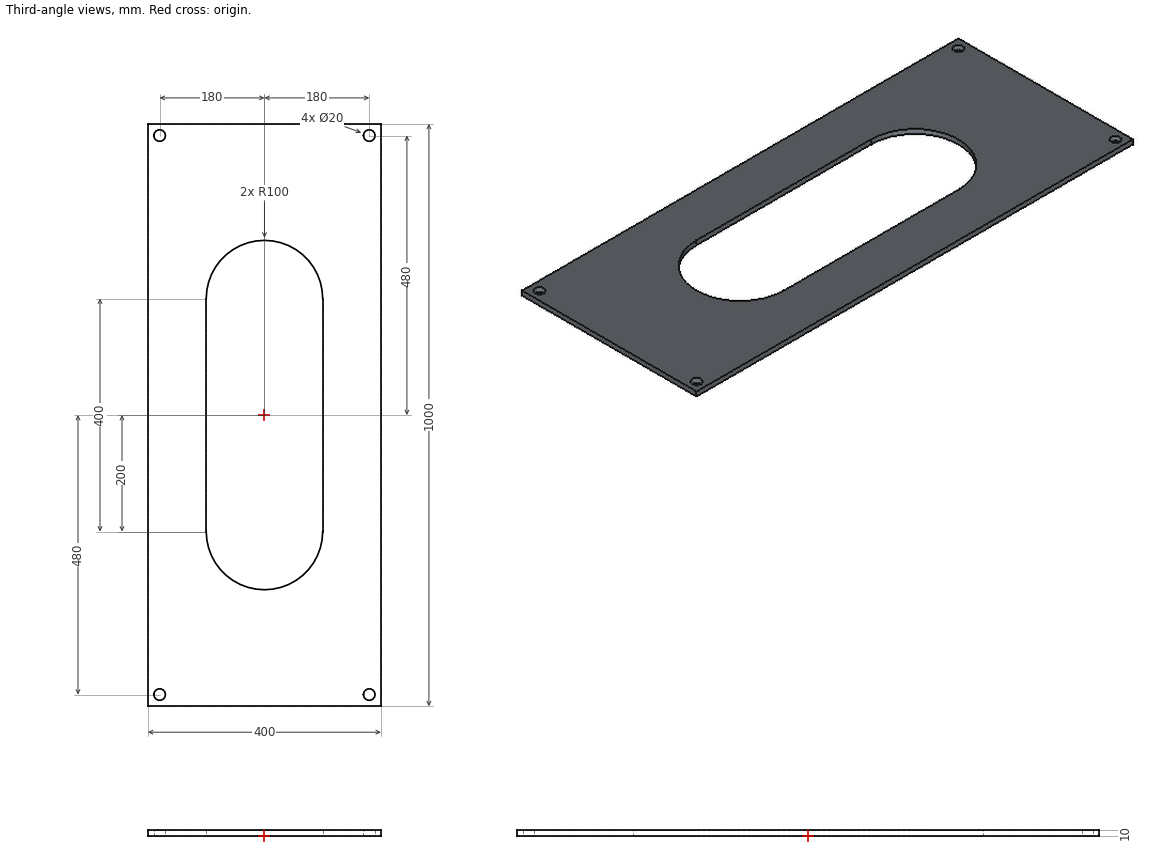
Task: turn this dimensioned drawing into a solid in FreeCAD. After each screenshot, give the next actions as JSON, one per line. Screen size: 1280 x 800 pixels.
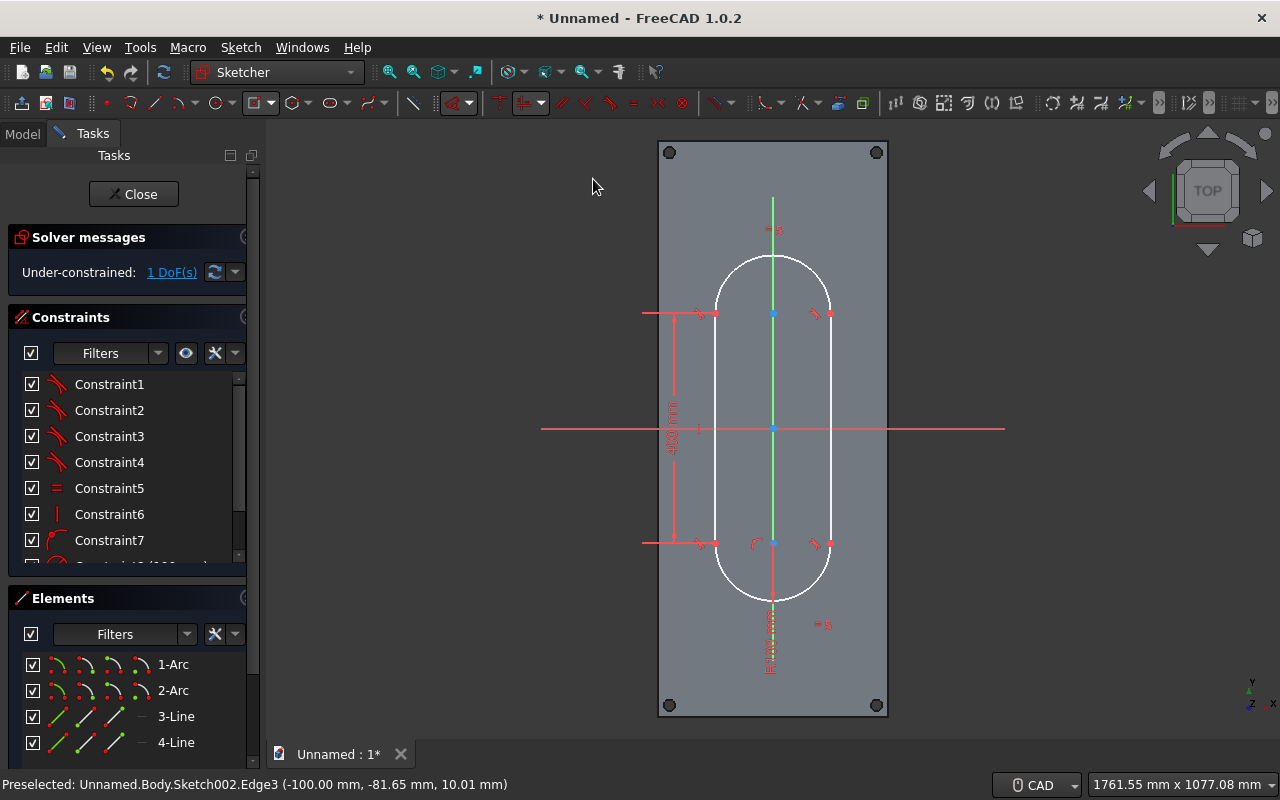
{"action": "left_click", "coordinate": [715, 543]}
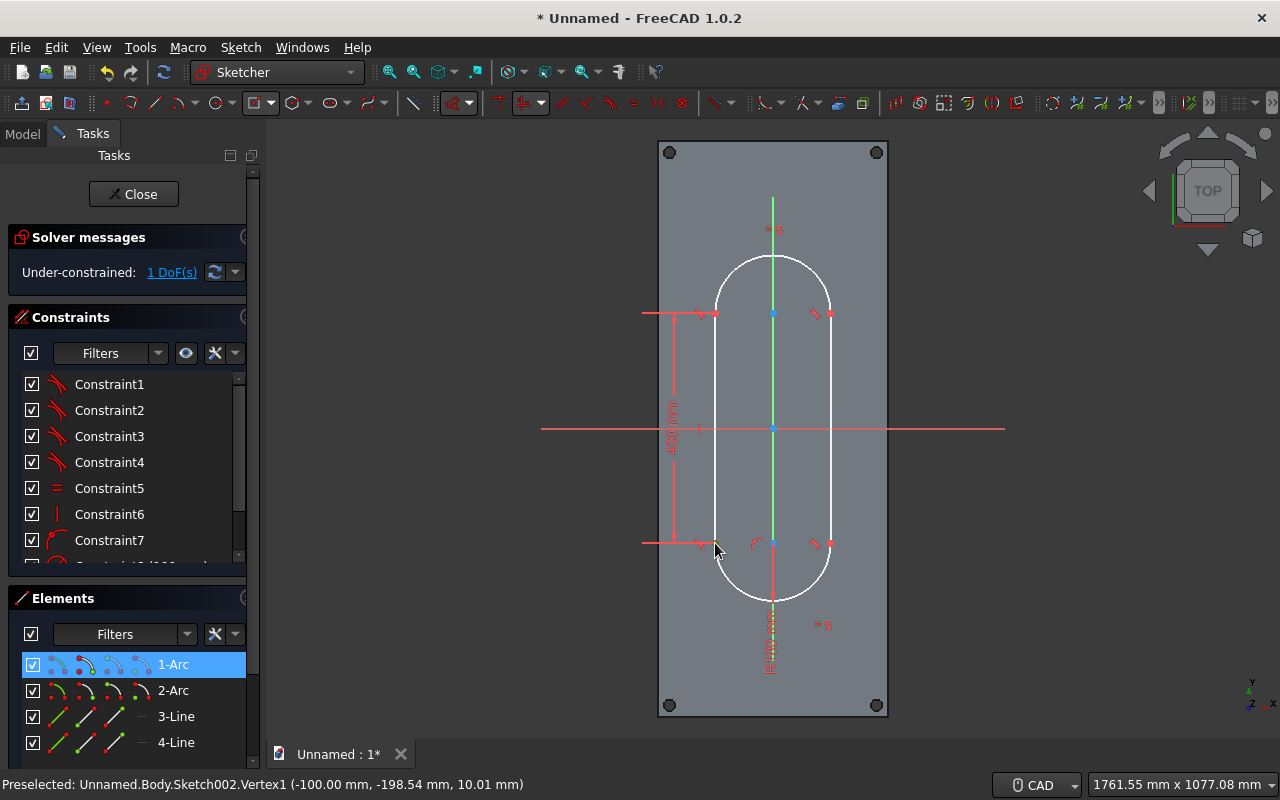
{"action": "left_click", "coordinate": [472, 104]}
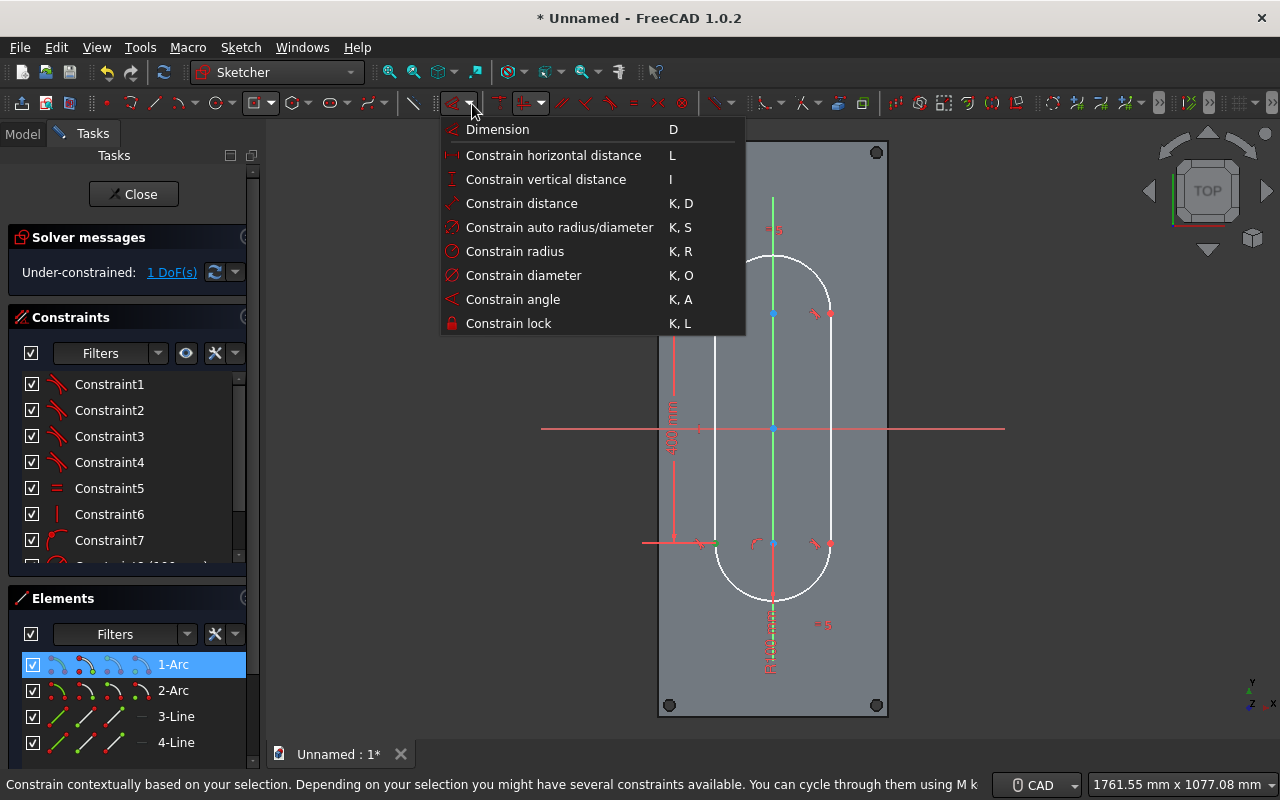
{"action": "left_click", "coordinate": [593, 179]}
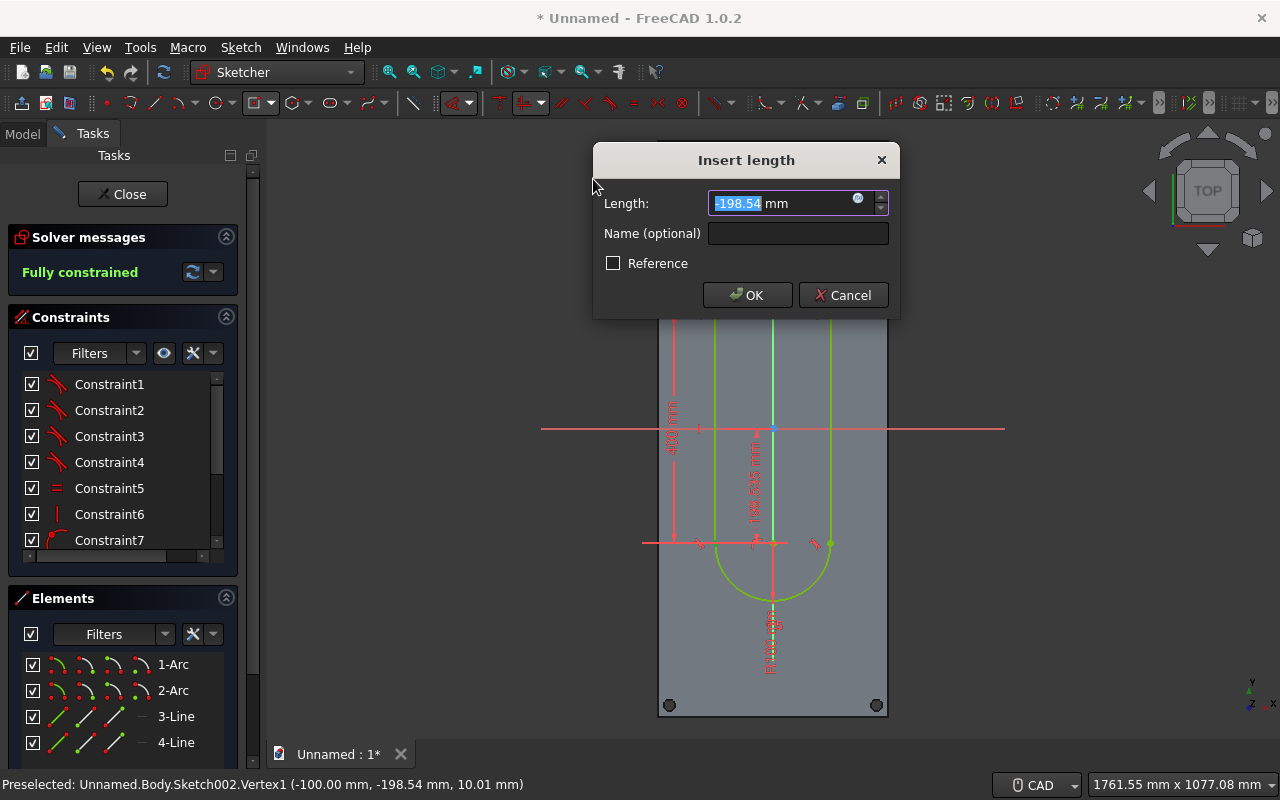
{"action": "type", "text": "-200"}
{"action": "key", "text": "Return"}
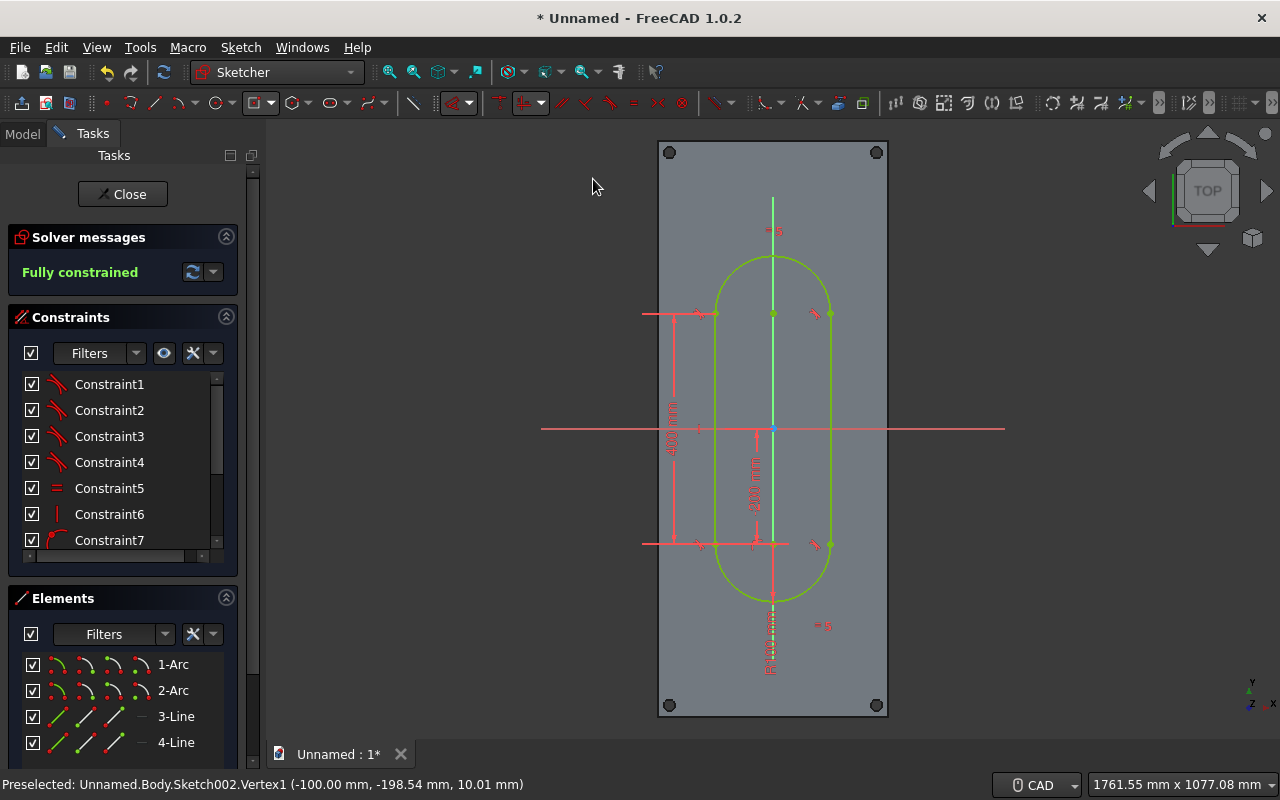
{"action": "left_click", "coordinate": [123, 194]}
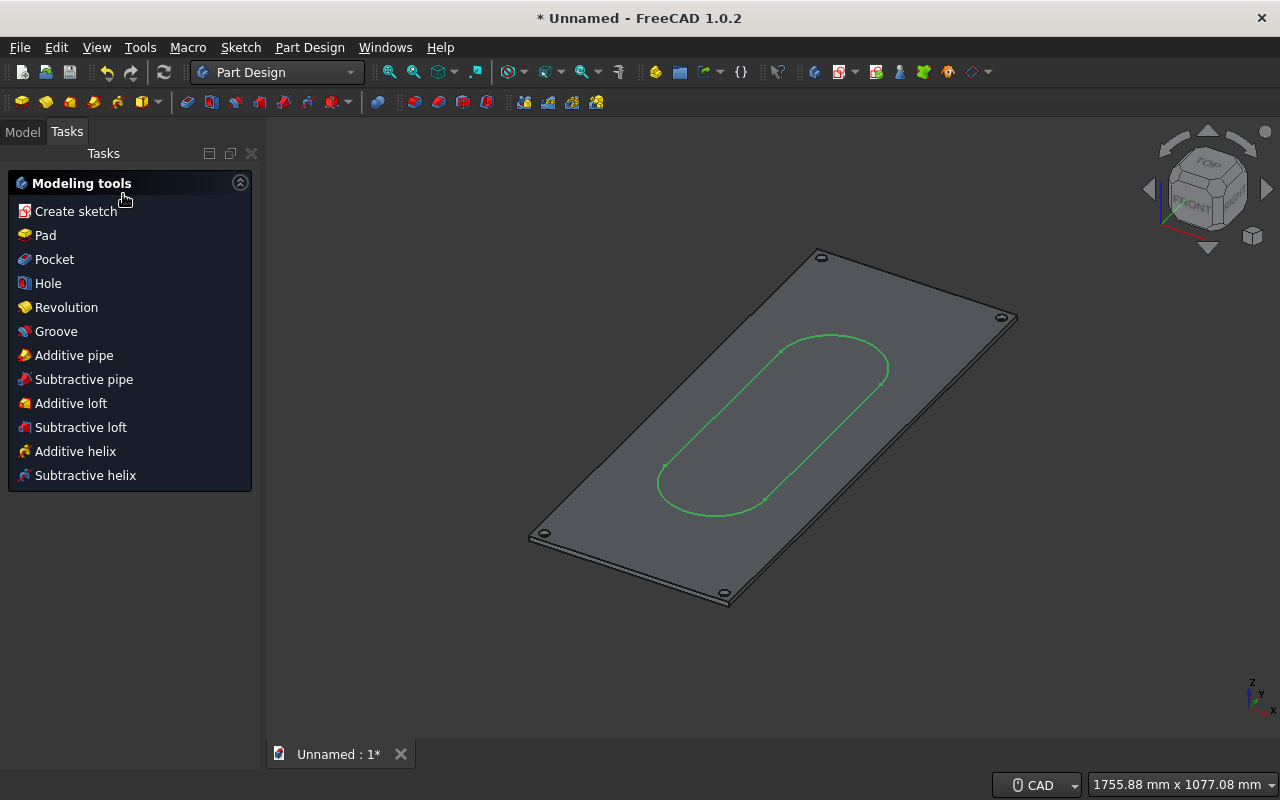
{"action": "left_click", "coordinate": [188, 102]}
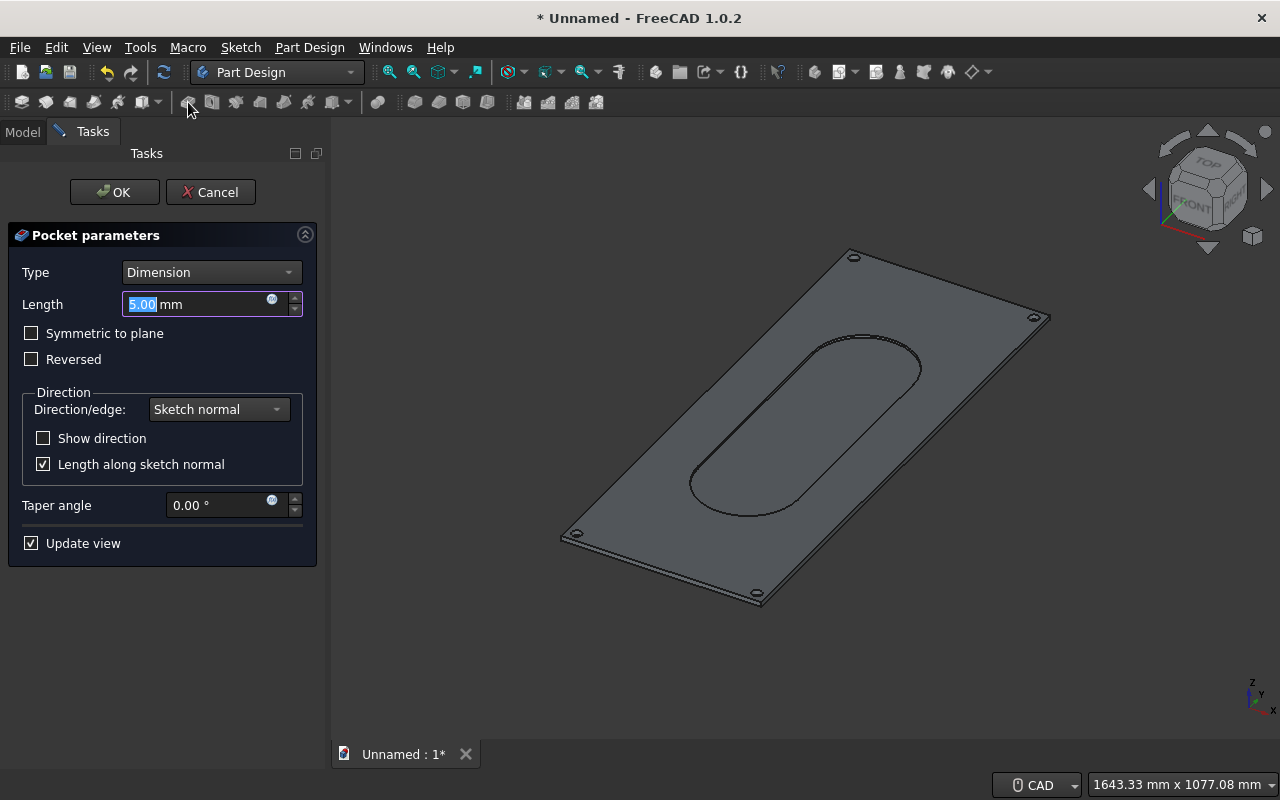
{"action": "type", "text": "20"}
{"action": "key", "text": "Tab"}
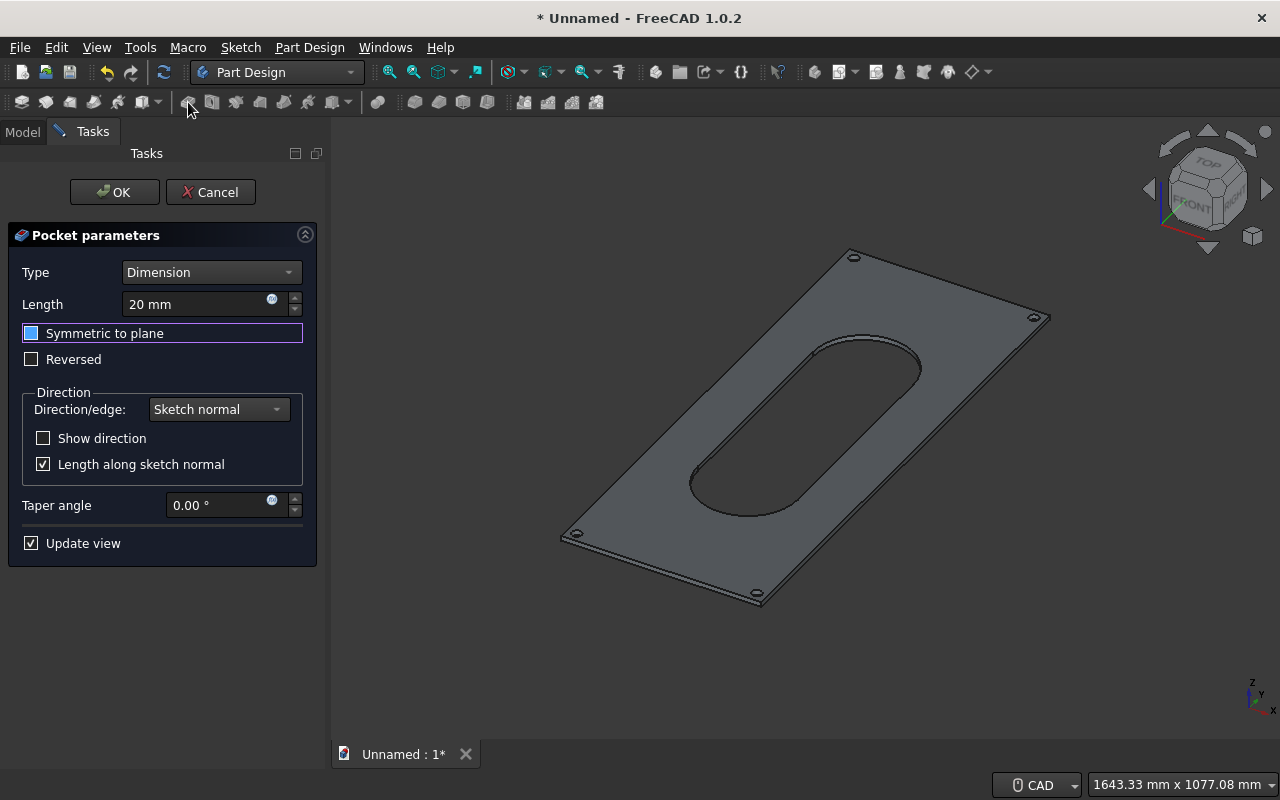
{"action": "left_click", "coordinate": [115, 192]}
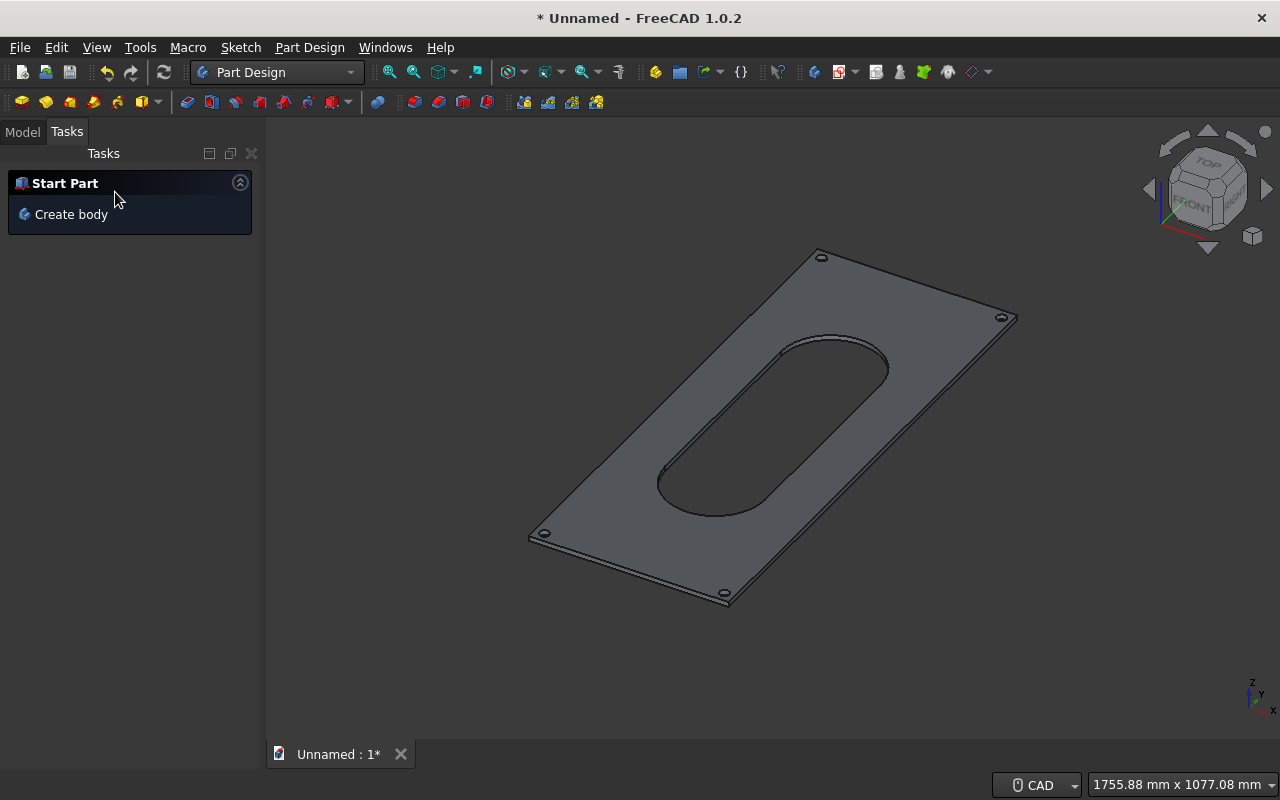
{"action": "key", "text": "0"}